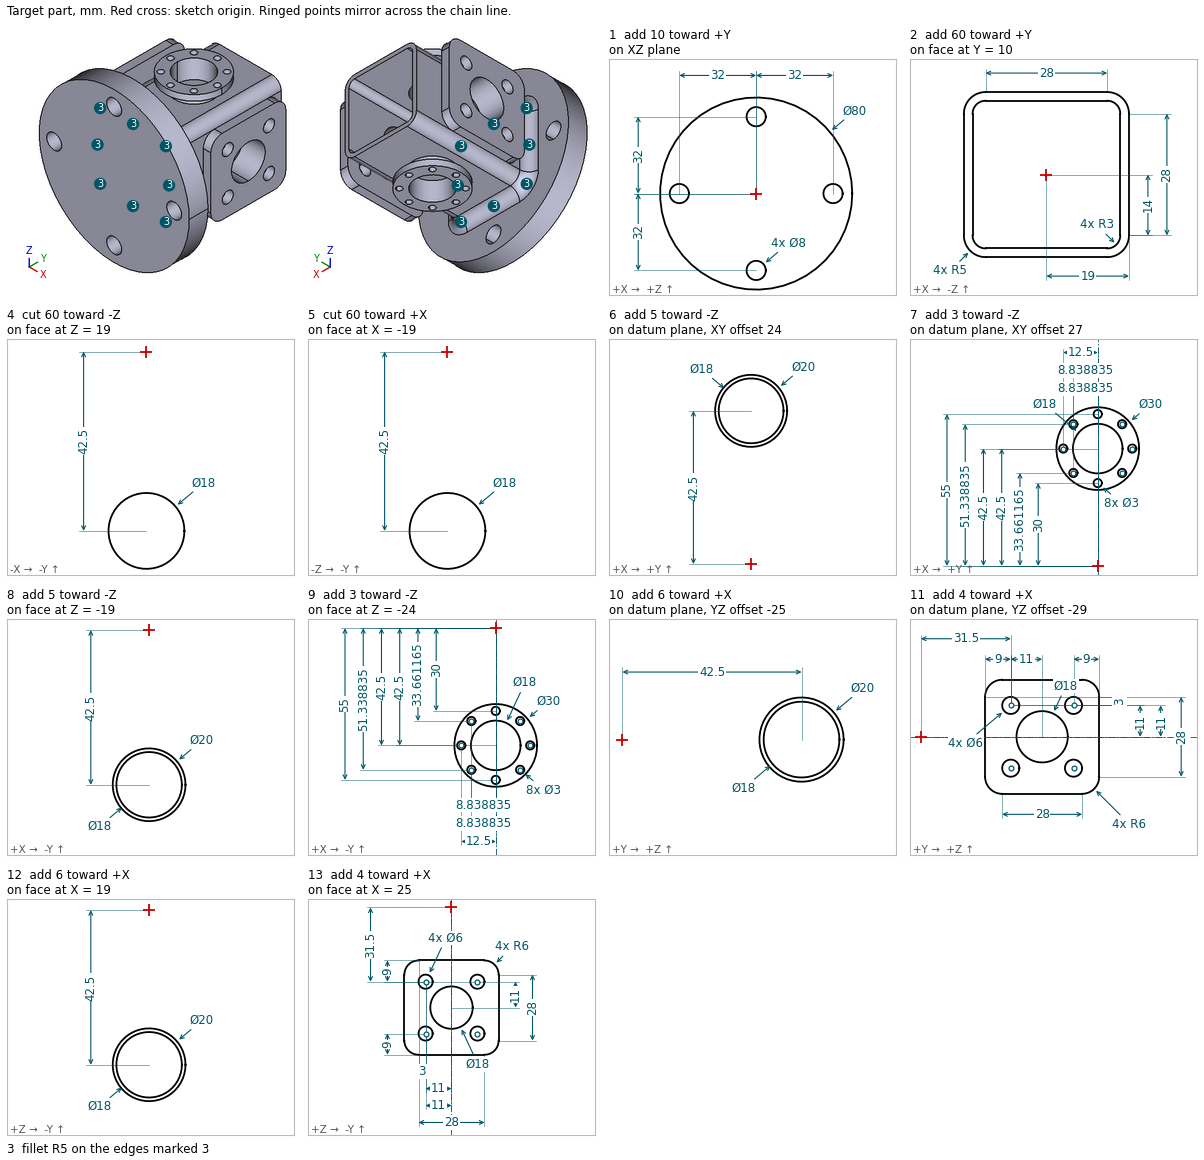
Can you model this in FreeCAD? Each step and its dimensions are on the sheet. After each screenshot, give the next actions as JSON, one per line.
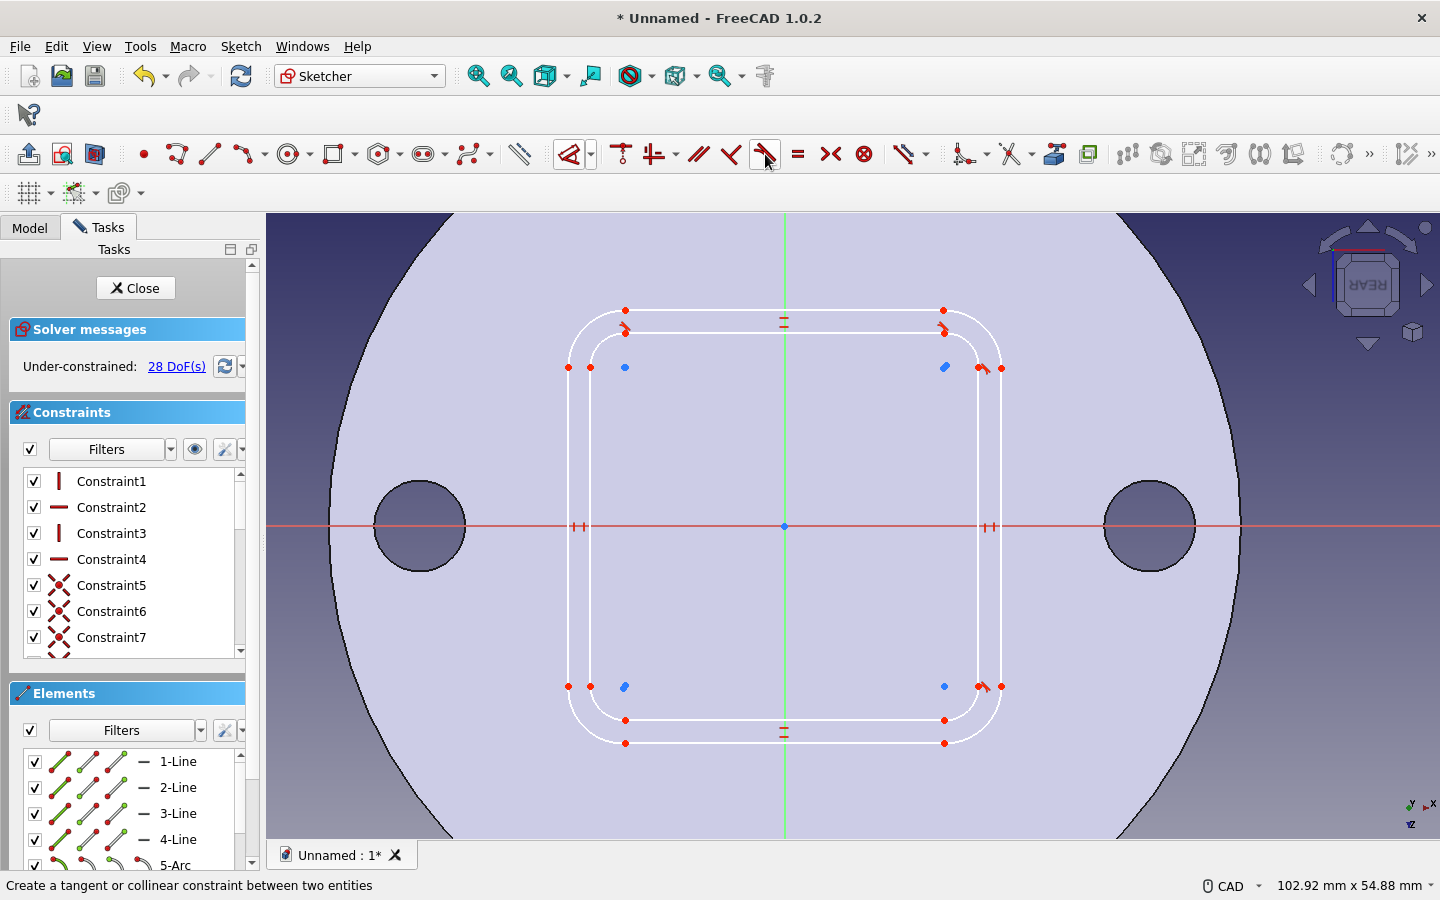
{"action": "left_click", "coordinate": [568, 463]}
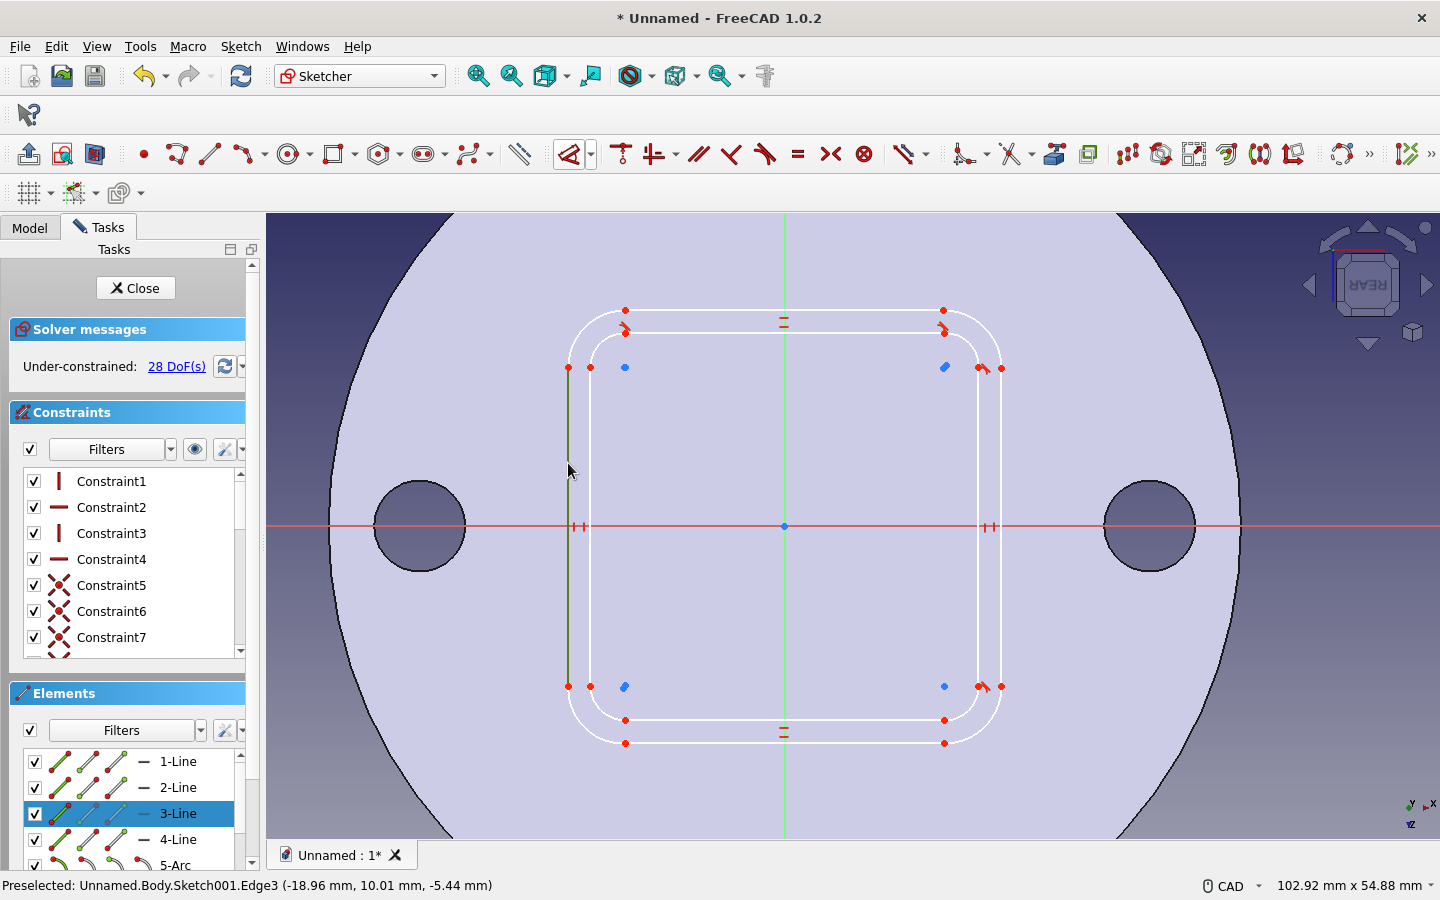
{"action": "left_click", "coordinate": [600, 317]}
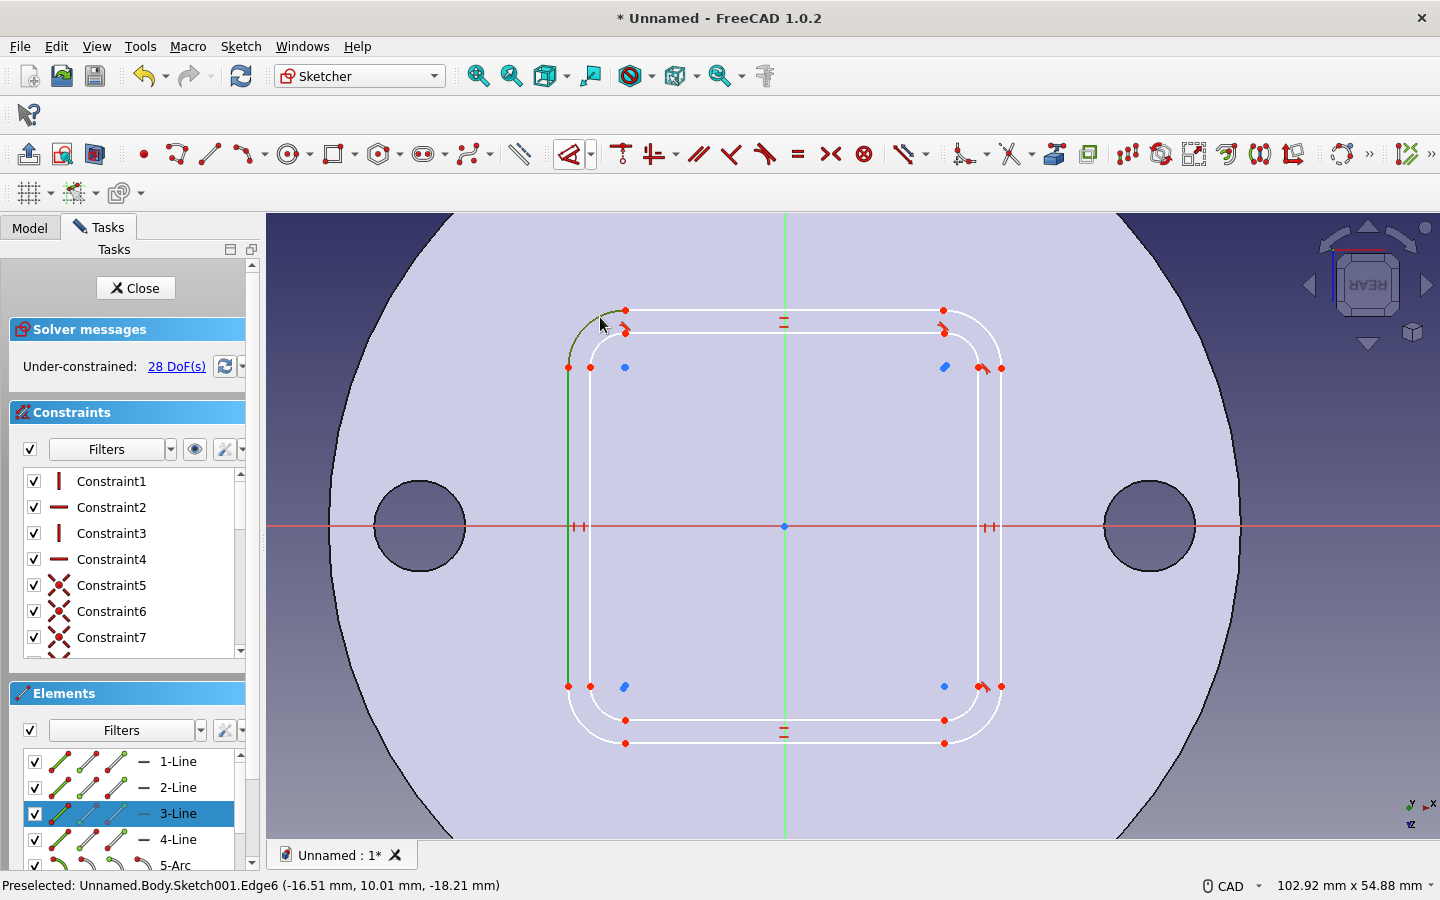
{"action": "key", "text": "t"}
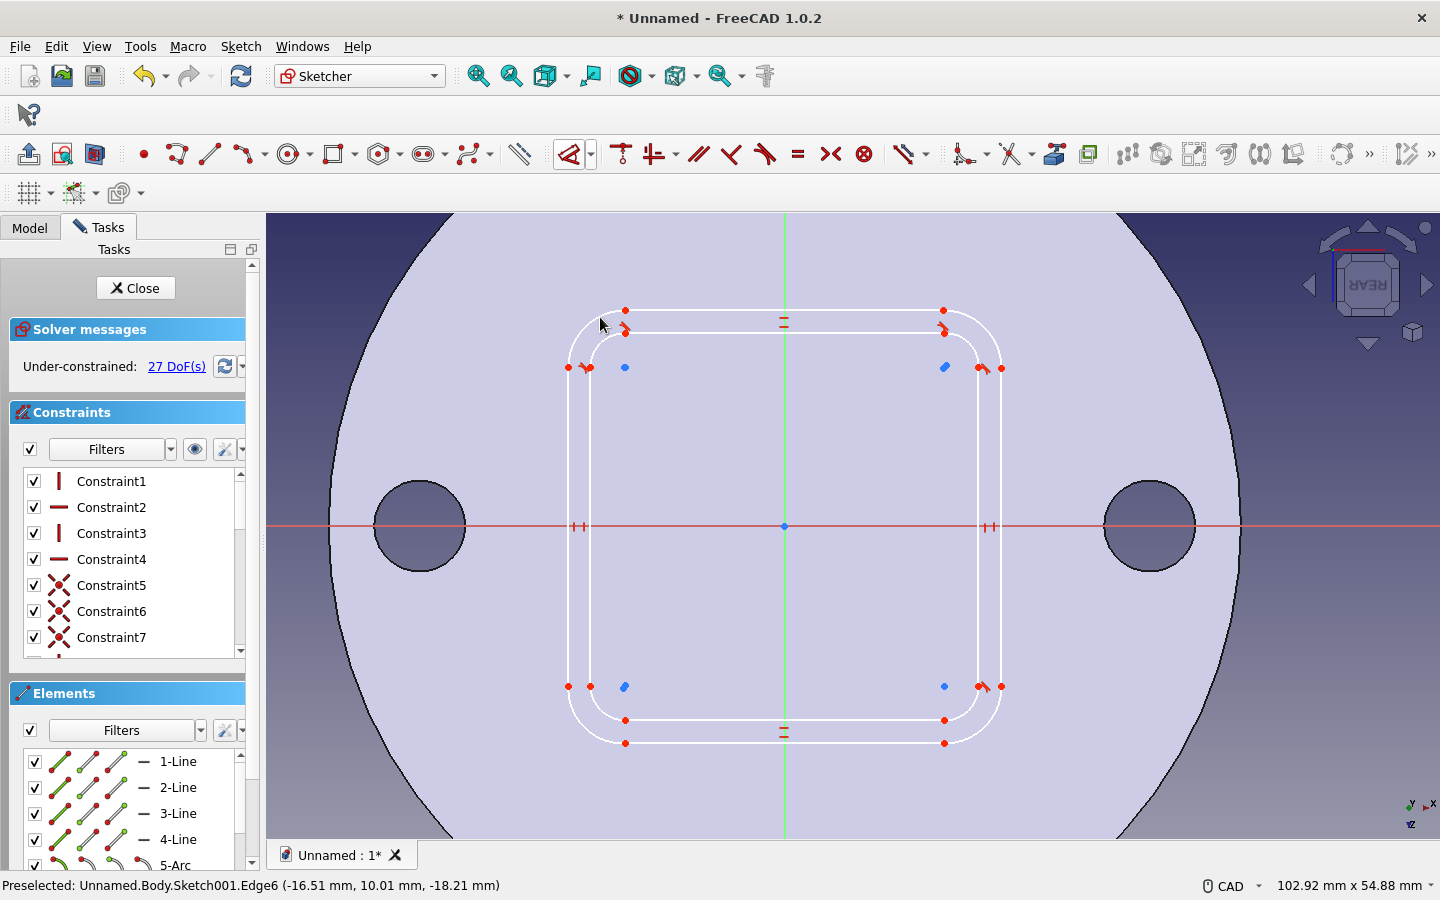
{"action": "left_click", "coordinate": [568, 463]}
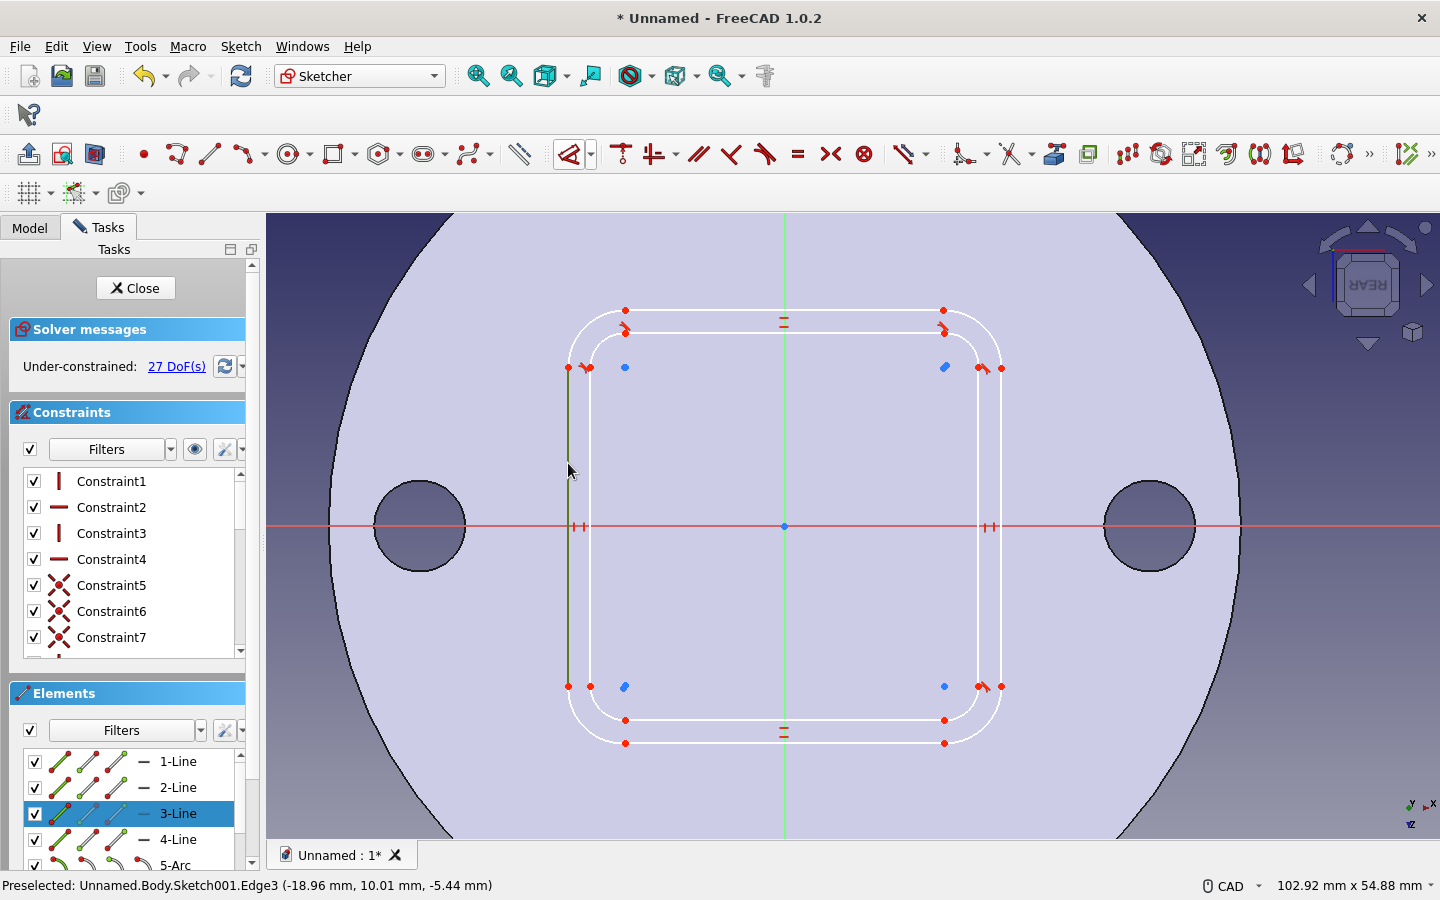
{"action": "left_click", "coordinate": [574, 713]}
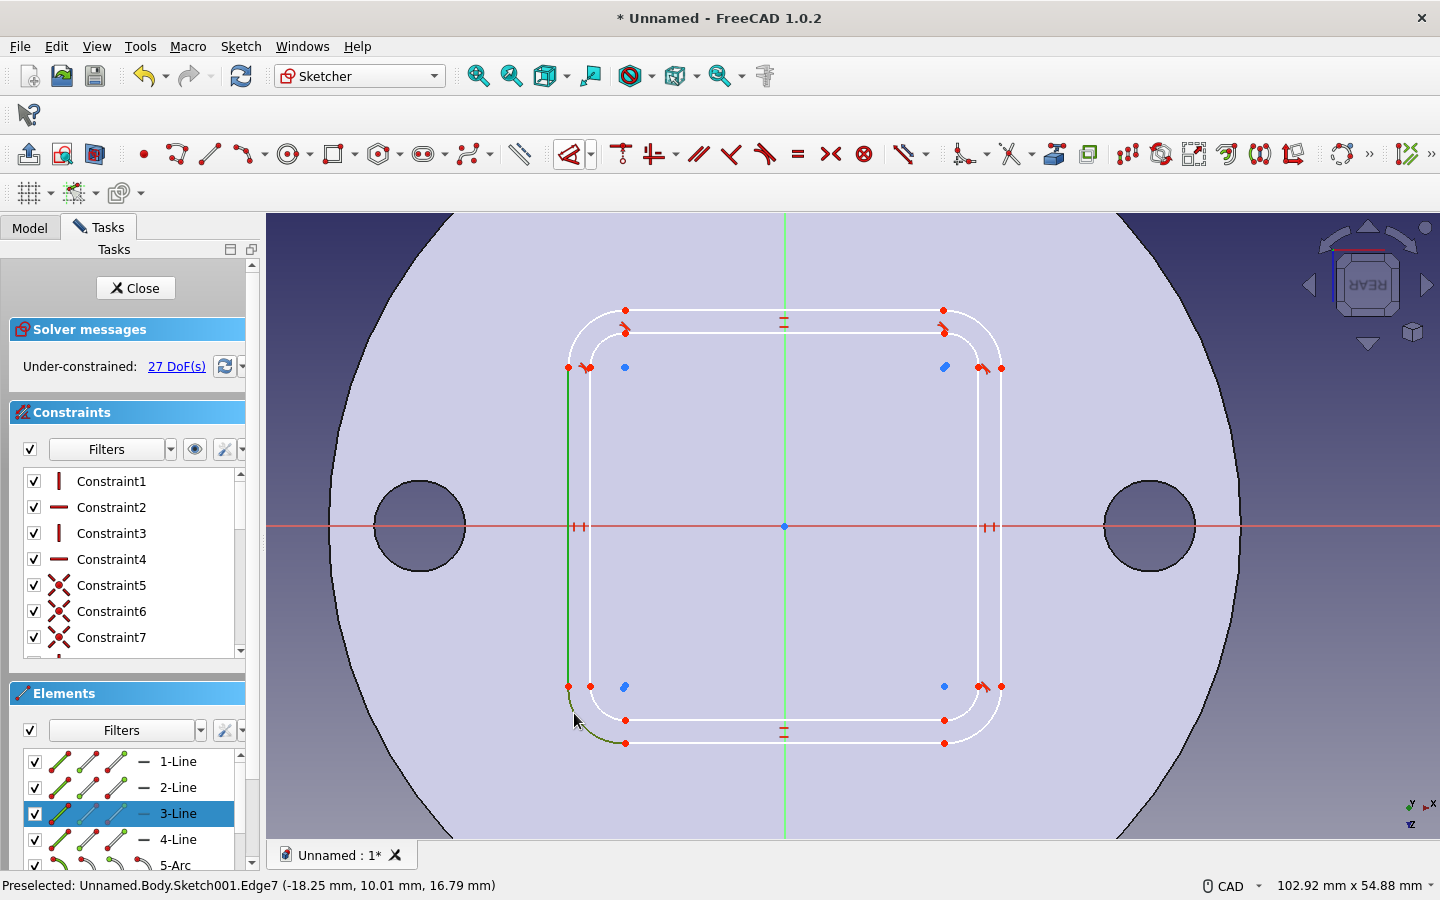
{"action": "key", "text": "t"}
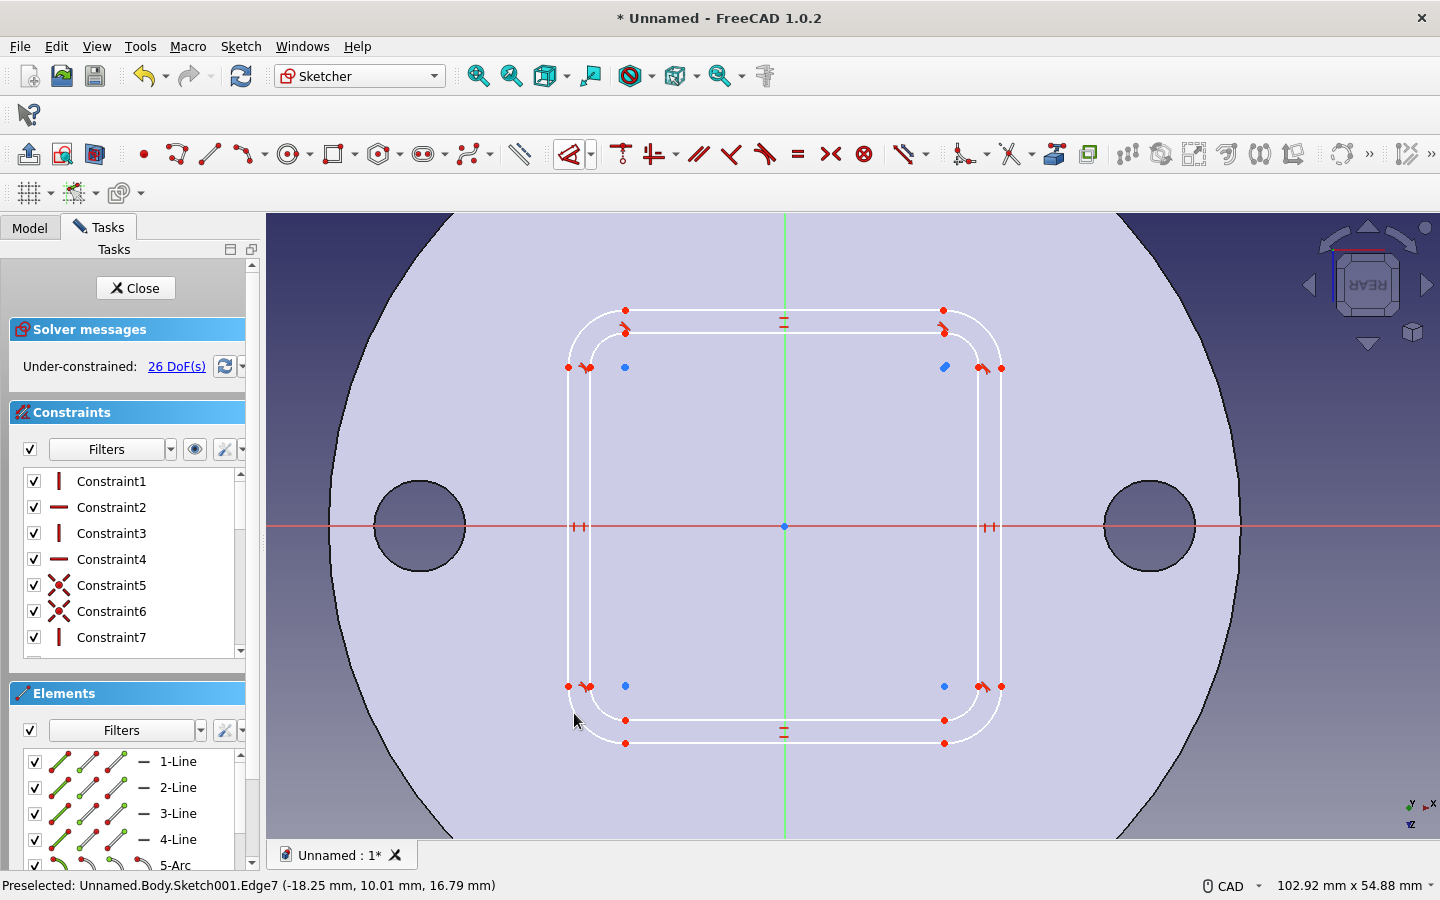
{"action": "left_click", "coordinate": [721, 743]}